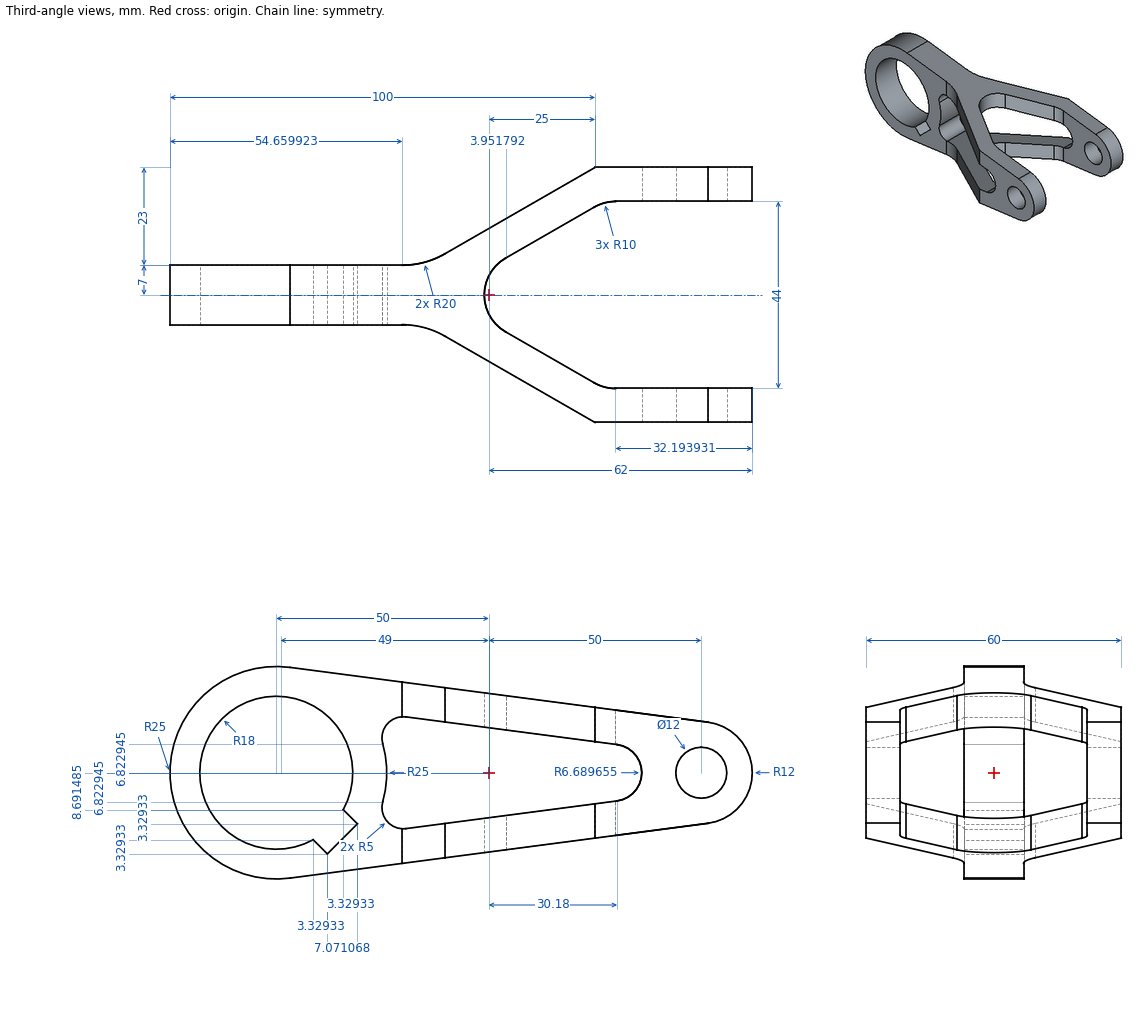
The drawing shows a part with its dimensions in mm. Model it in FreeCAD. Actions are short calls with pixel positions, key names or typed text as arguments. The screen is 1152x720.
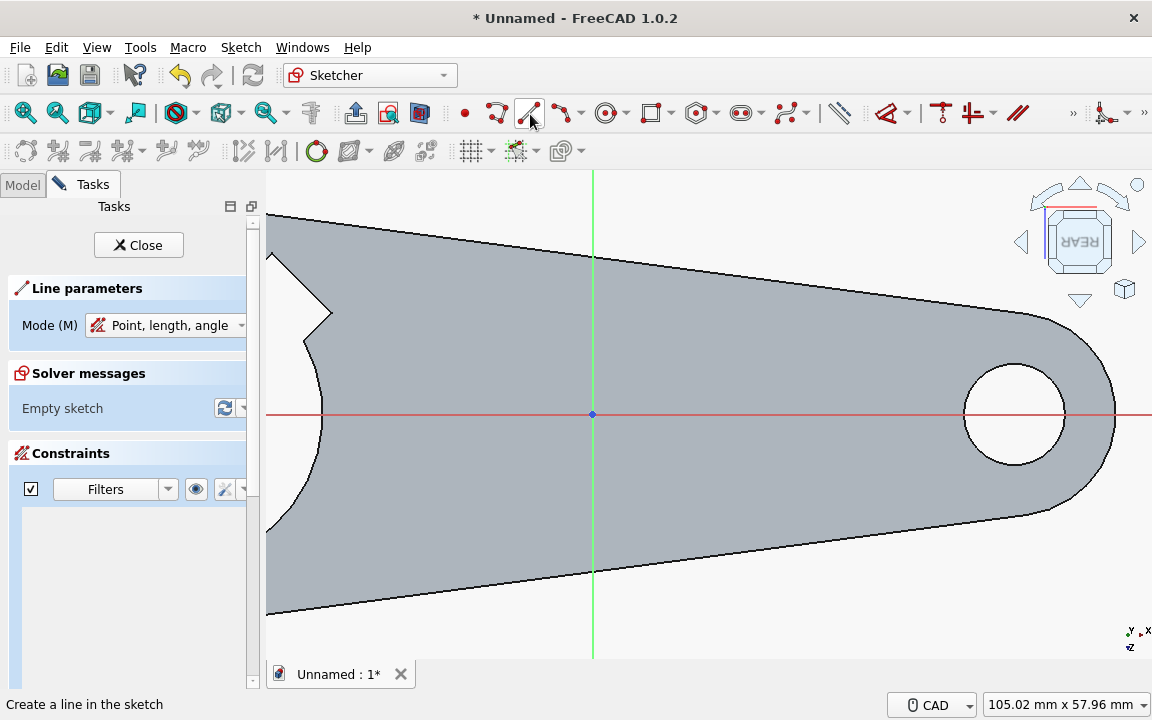
click(847, 359)
click(428, 304)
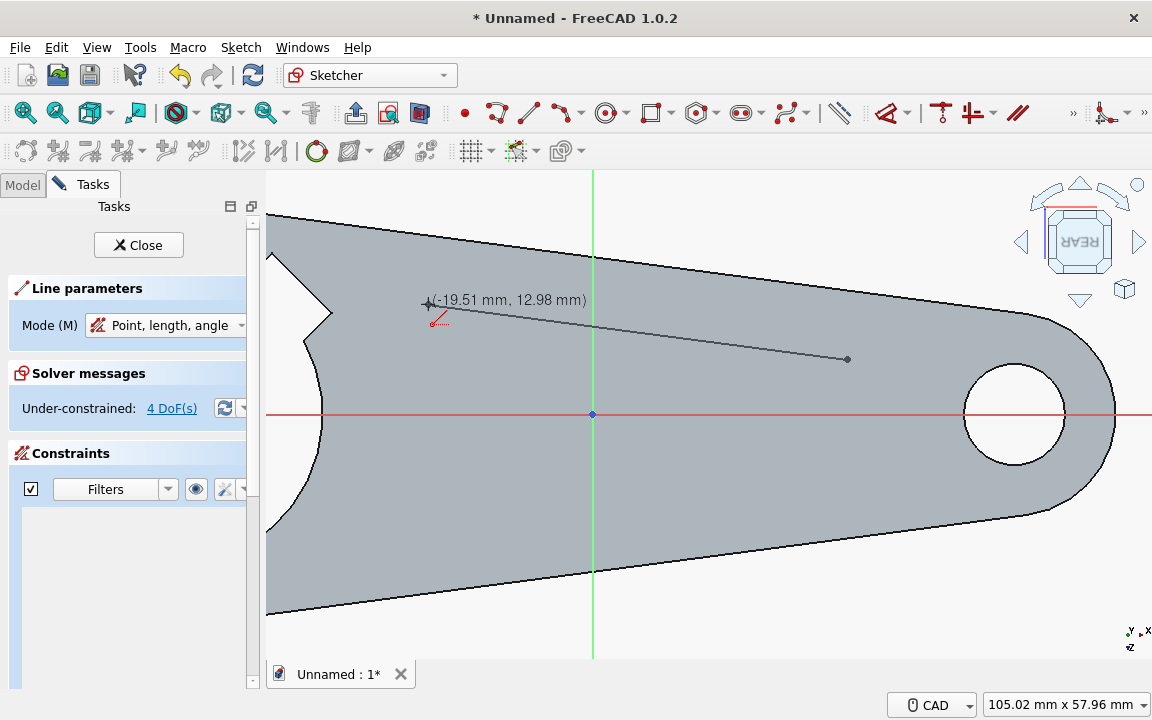
click(428, 525)
click(847, 470)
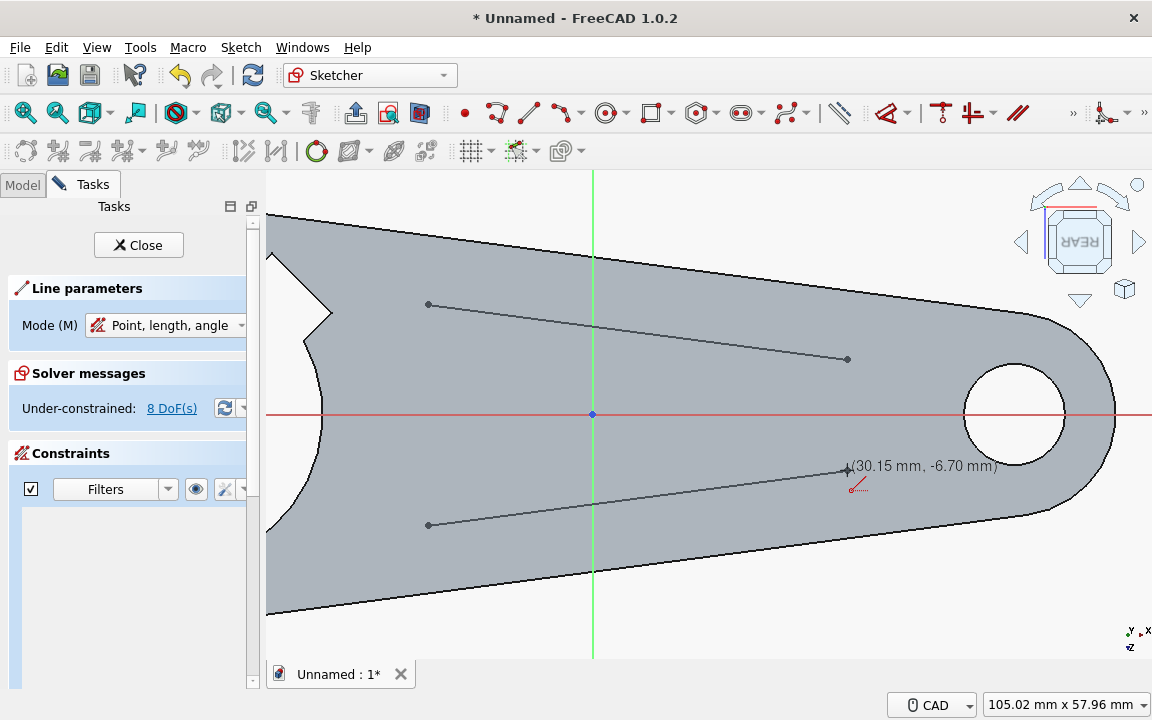
click(562, 114)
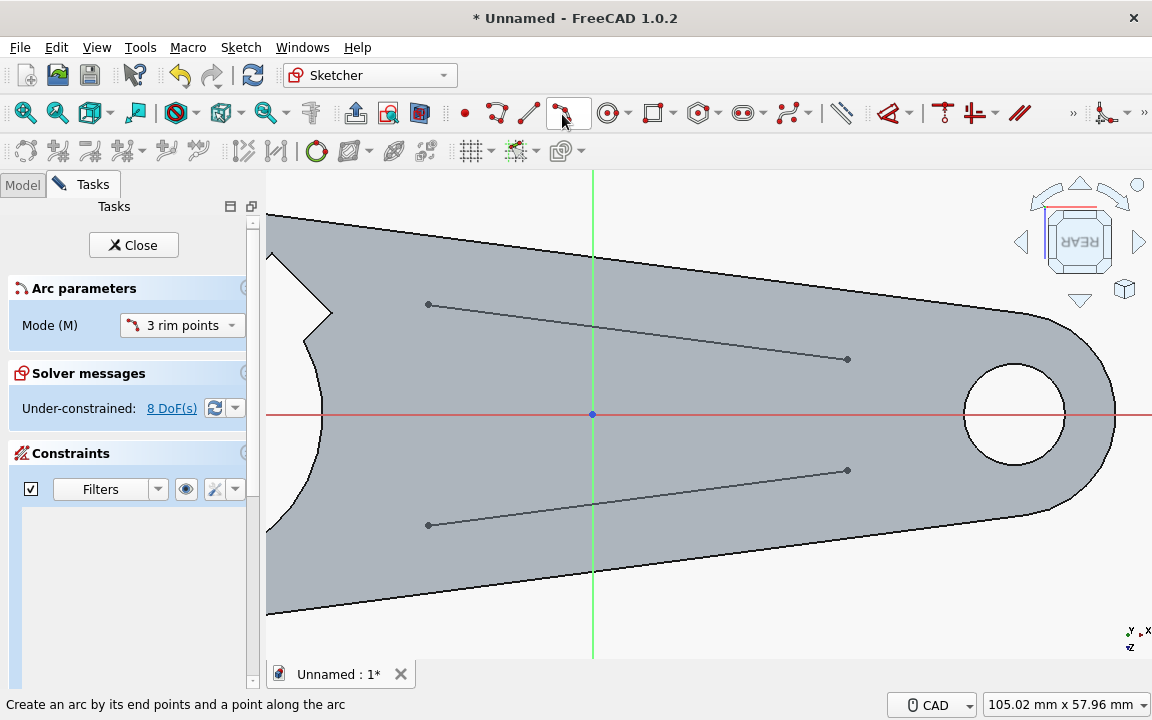
click(428, 305)
click(382, 357)
click(391, 318)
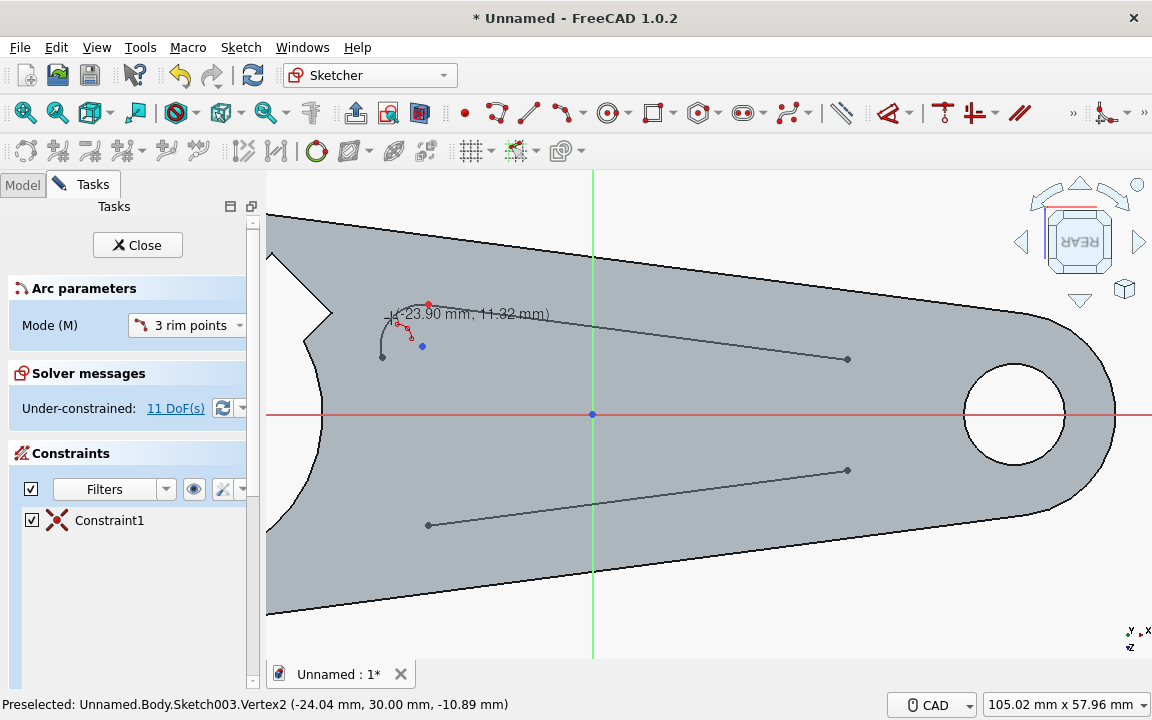
click(382, 358)
click(382, 472)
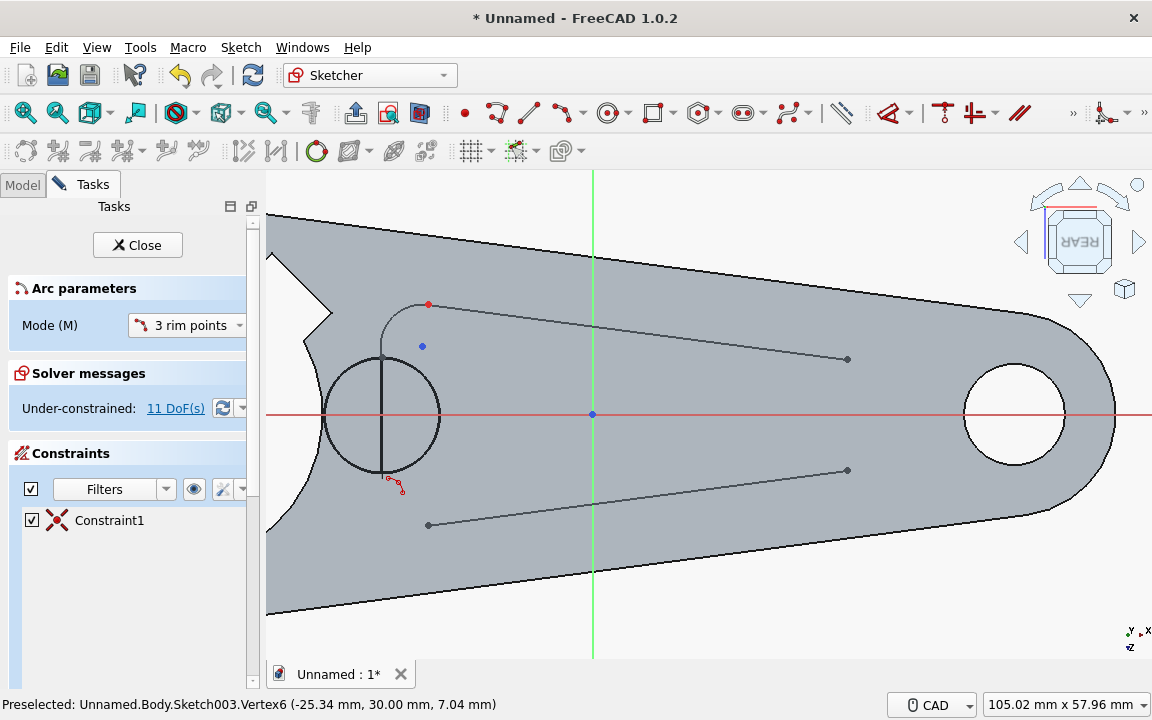
scroll(390, 426, up, 4)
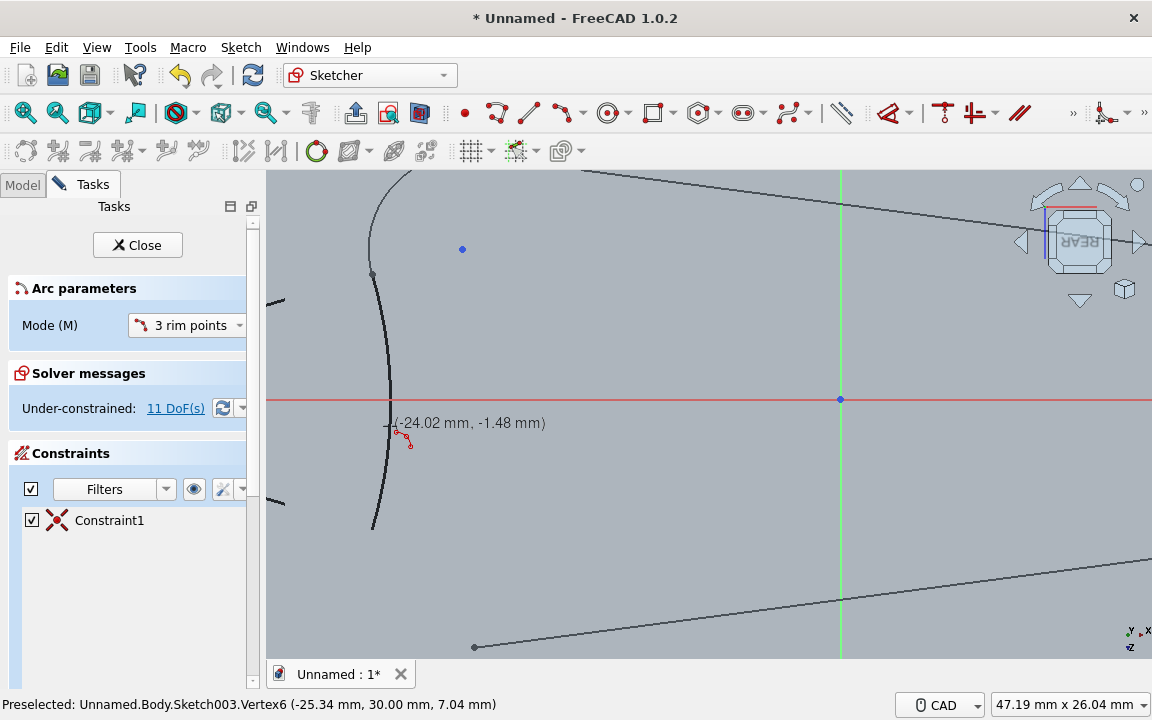
click(389, 426)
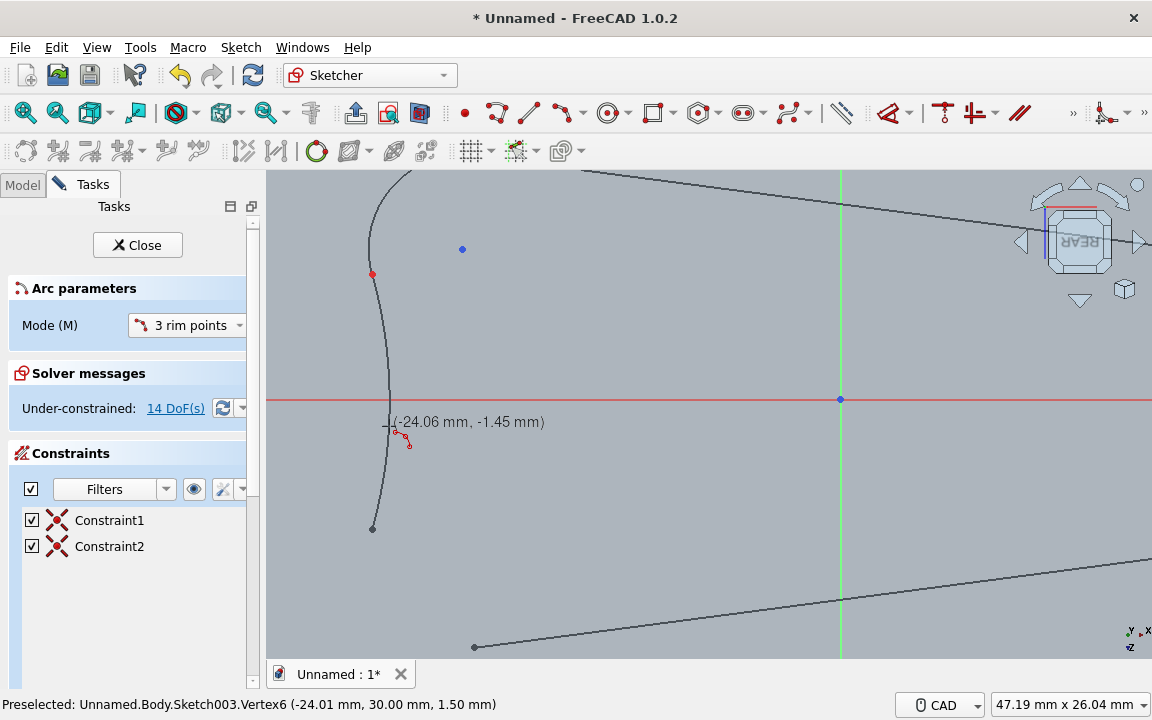
click(372, 530)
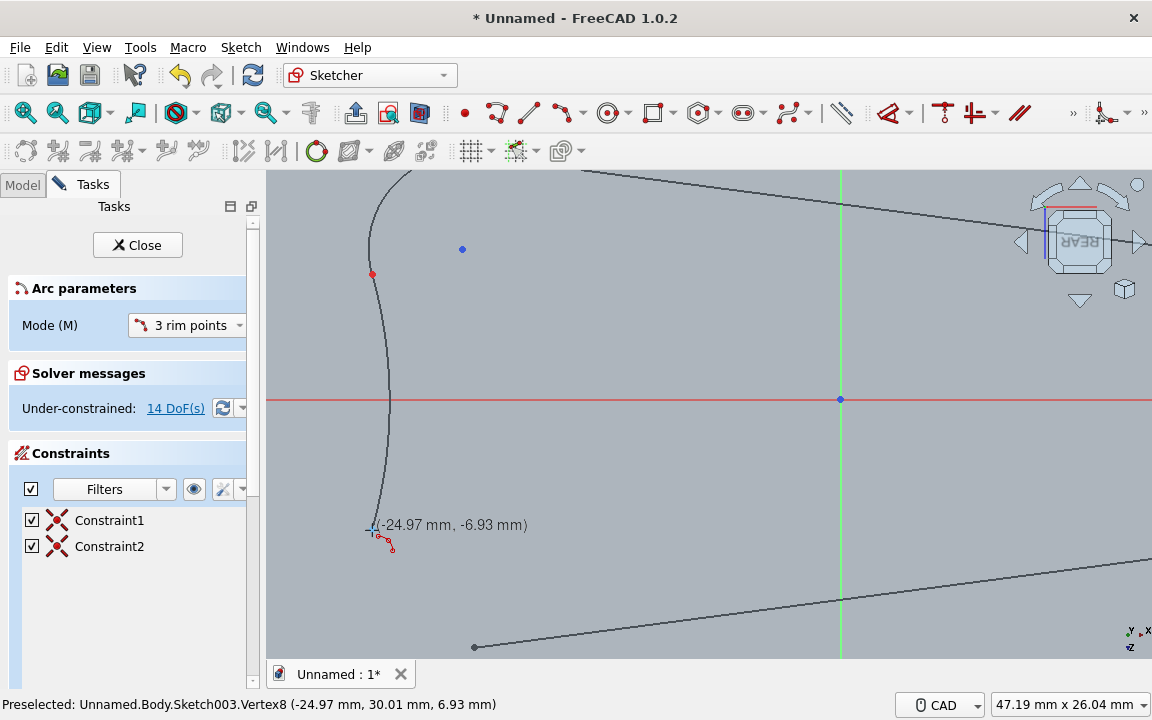
scroll(392, 427, down, 4)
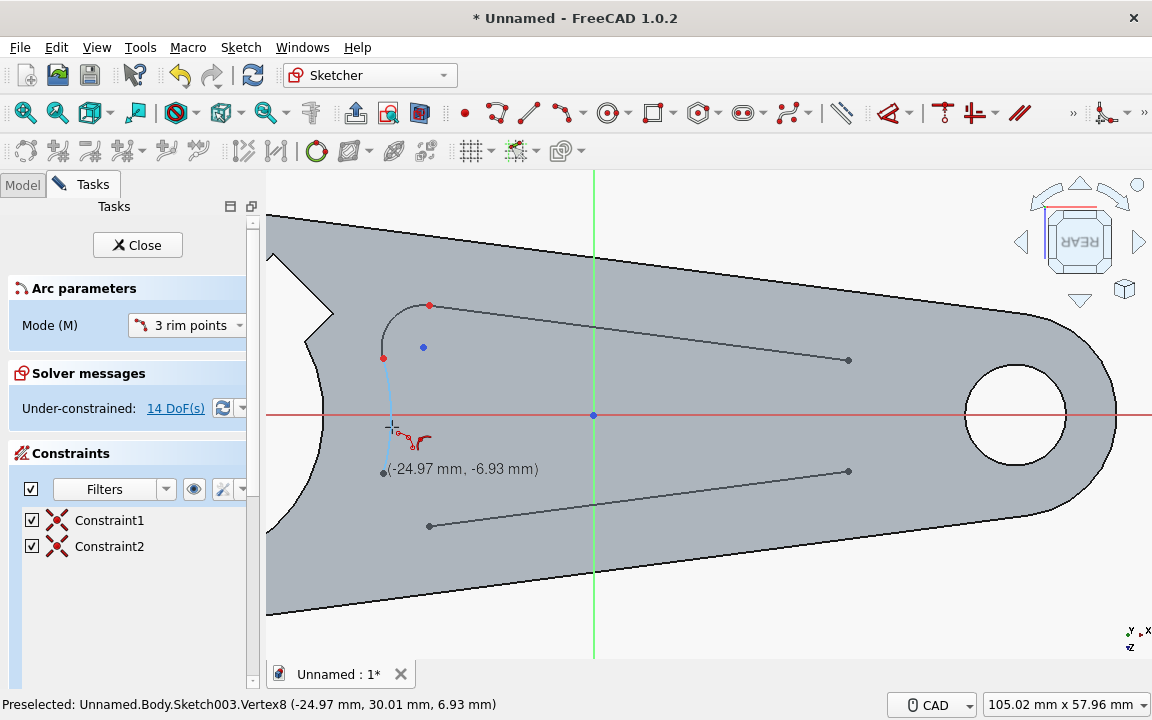
click(429, 527)
click(392, 512)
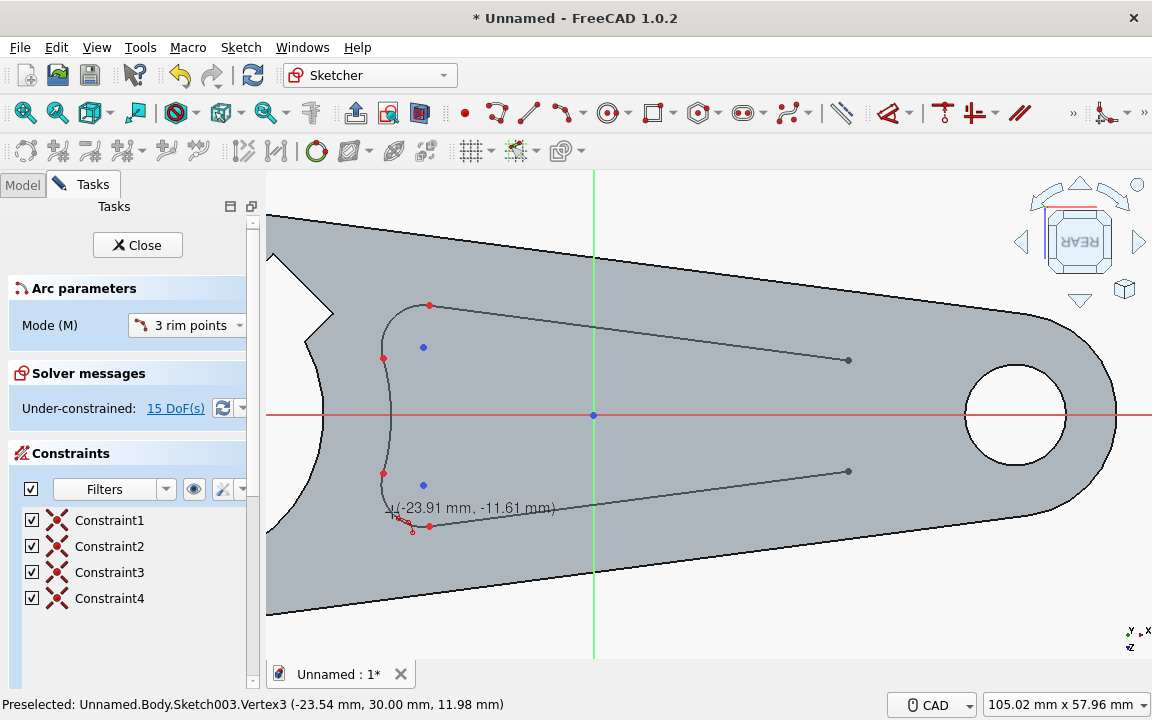
click(848, 472)
click(848, 361)
click(895, 431)
key(Escape)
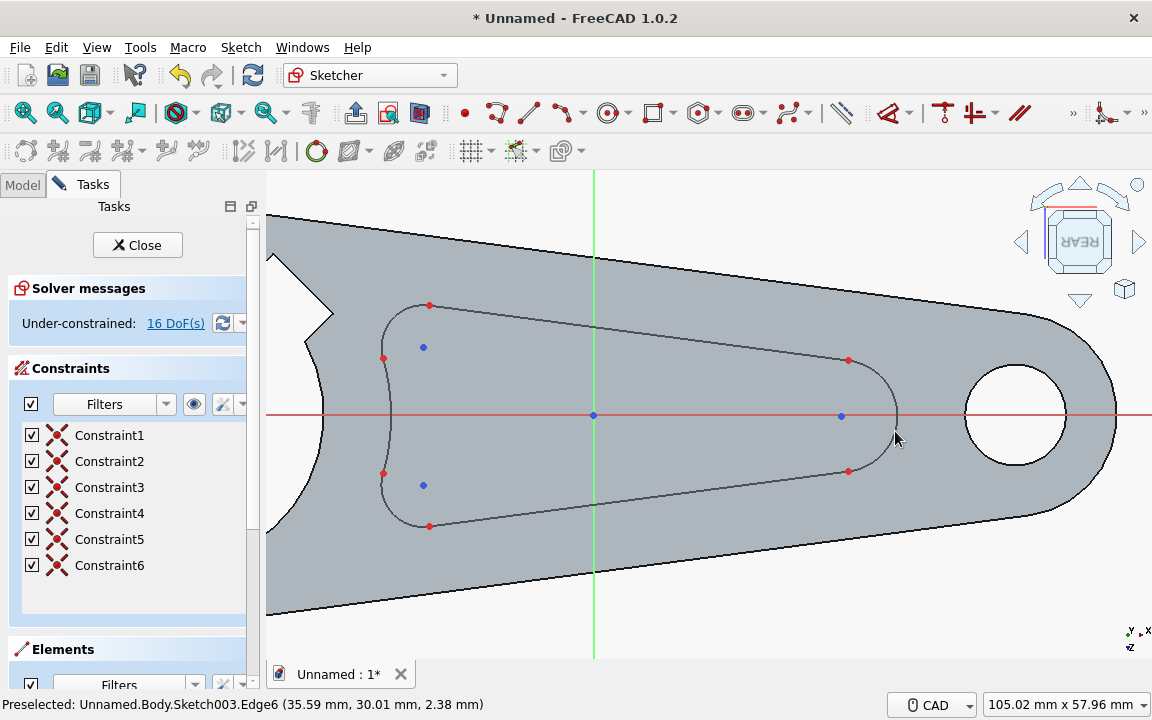
click(722, 344)